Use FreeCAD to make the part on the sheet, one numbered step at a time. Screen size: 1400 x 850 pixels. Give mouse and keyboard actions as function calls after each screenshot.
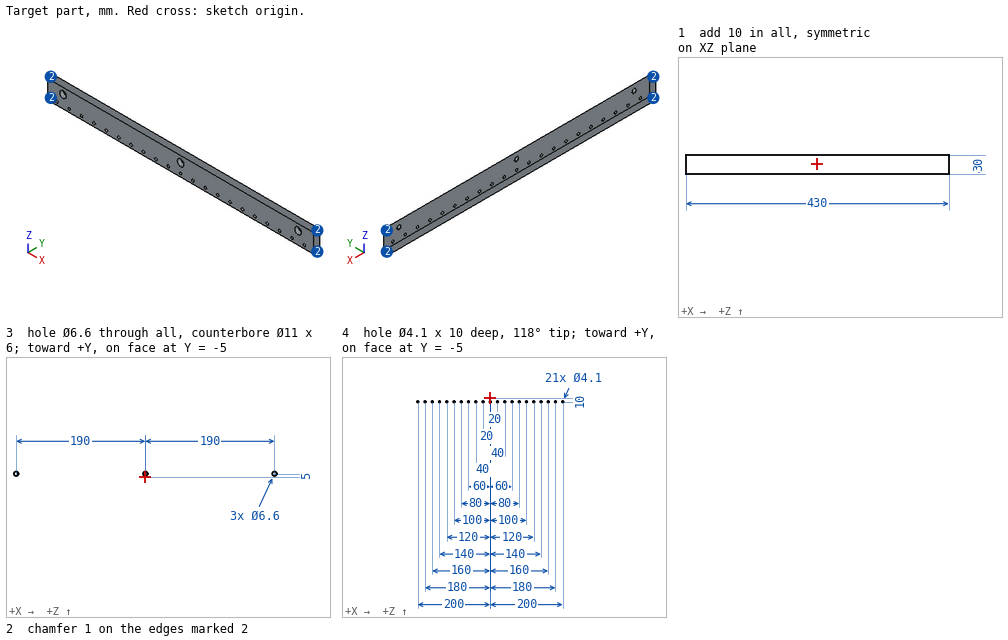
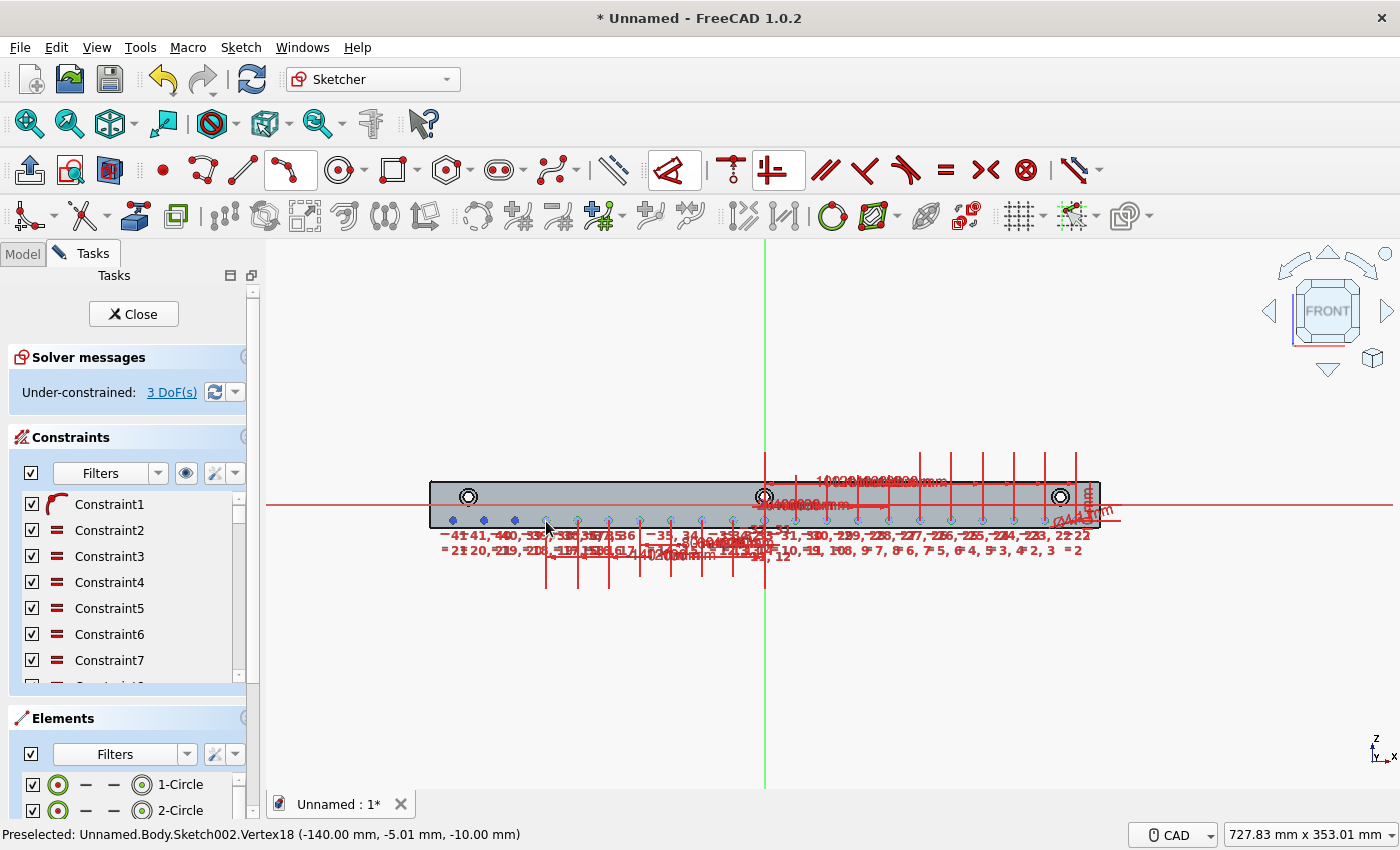
click(515, 521)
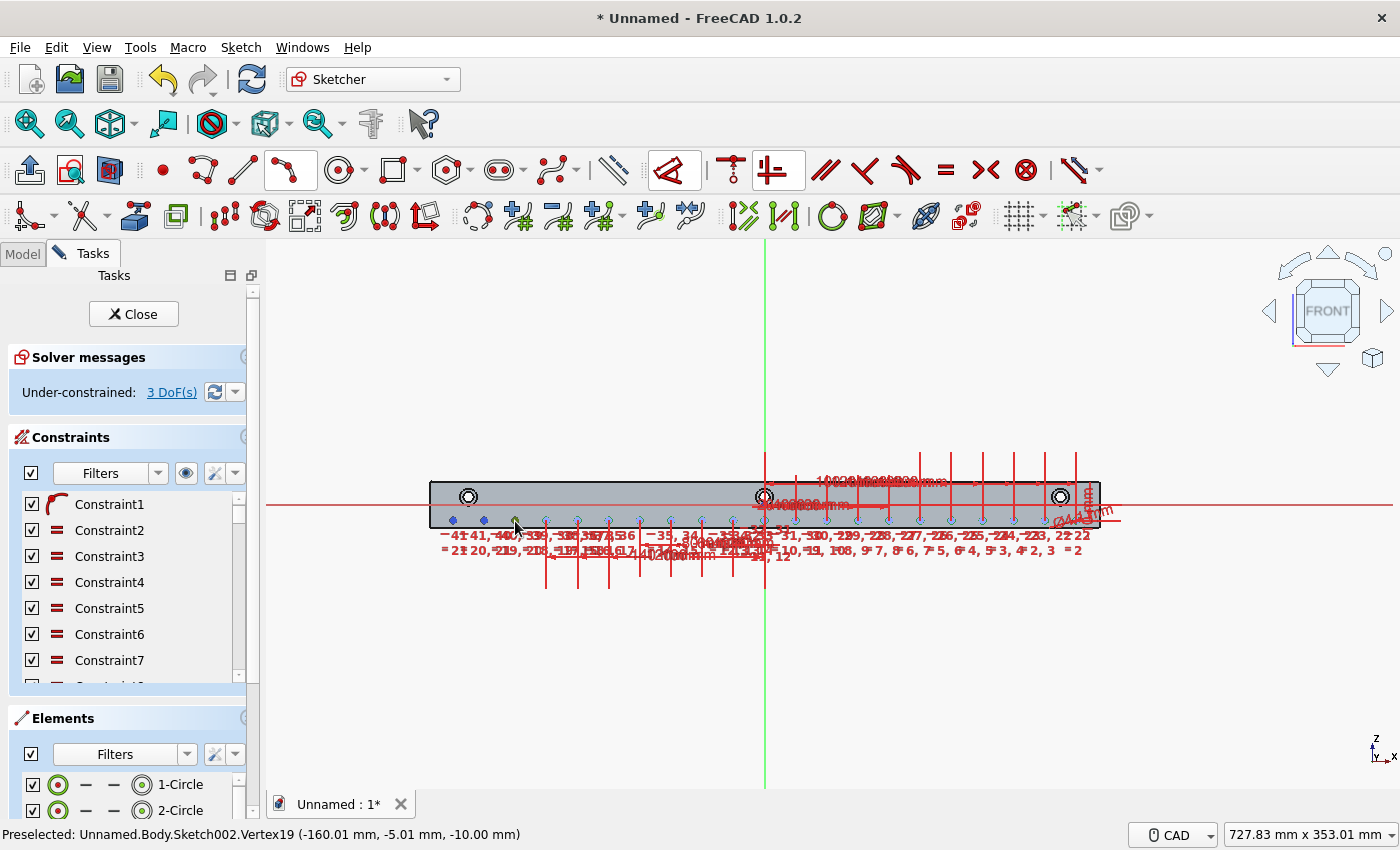
key(l)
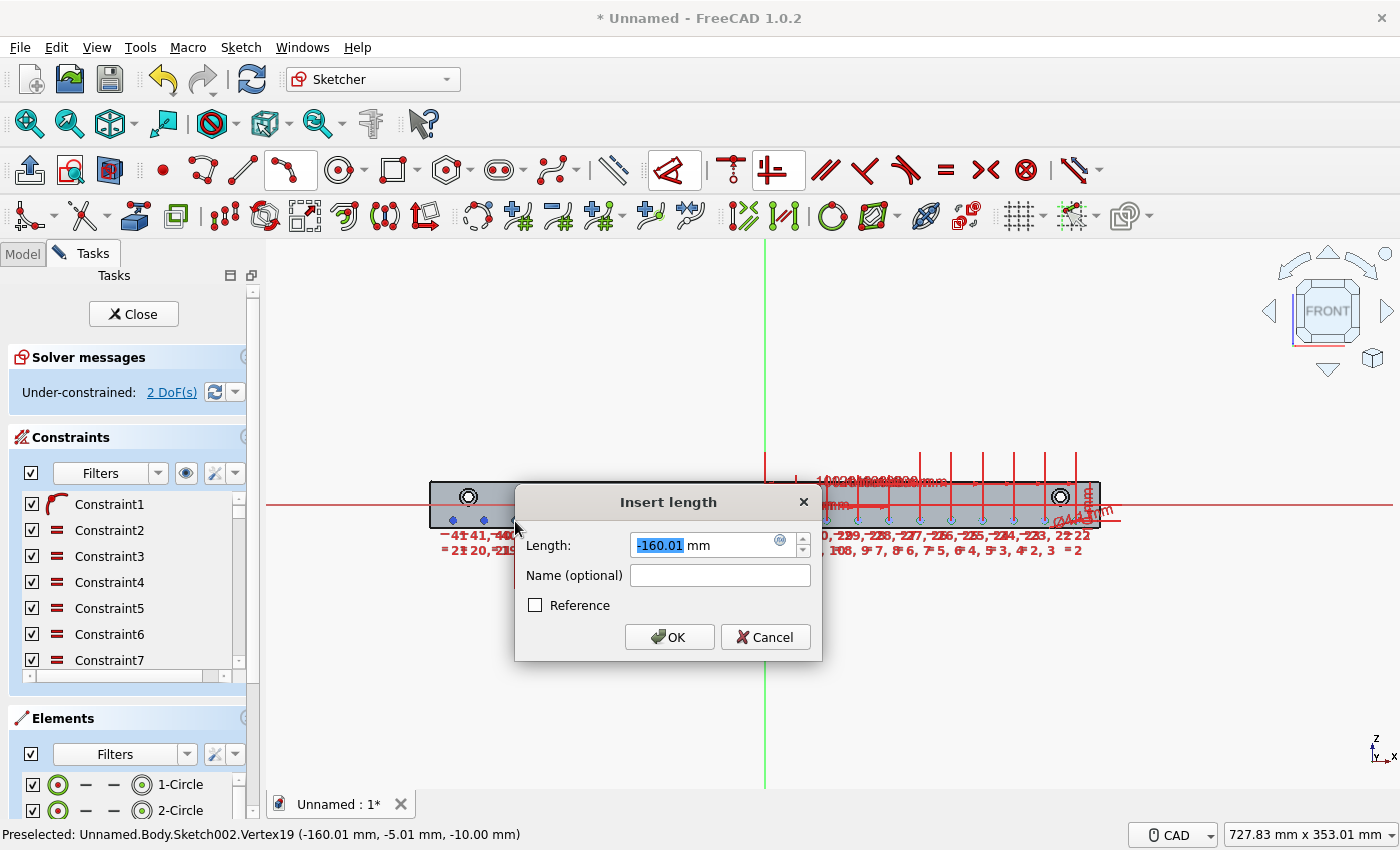
text(-160)
key(Return)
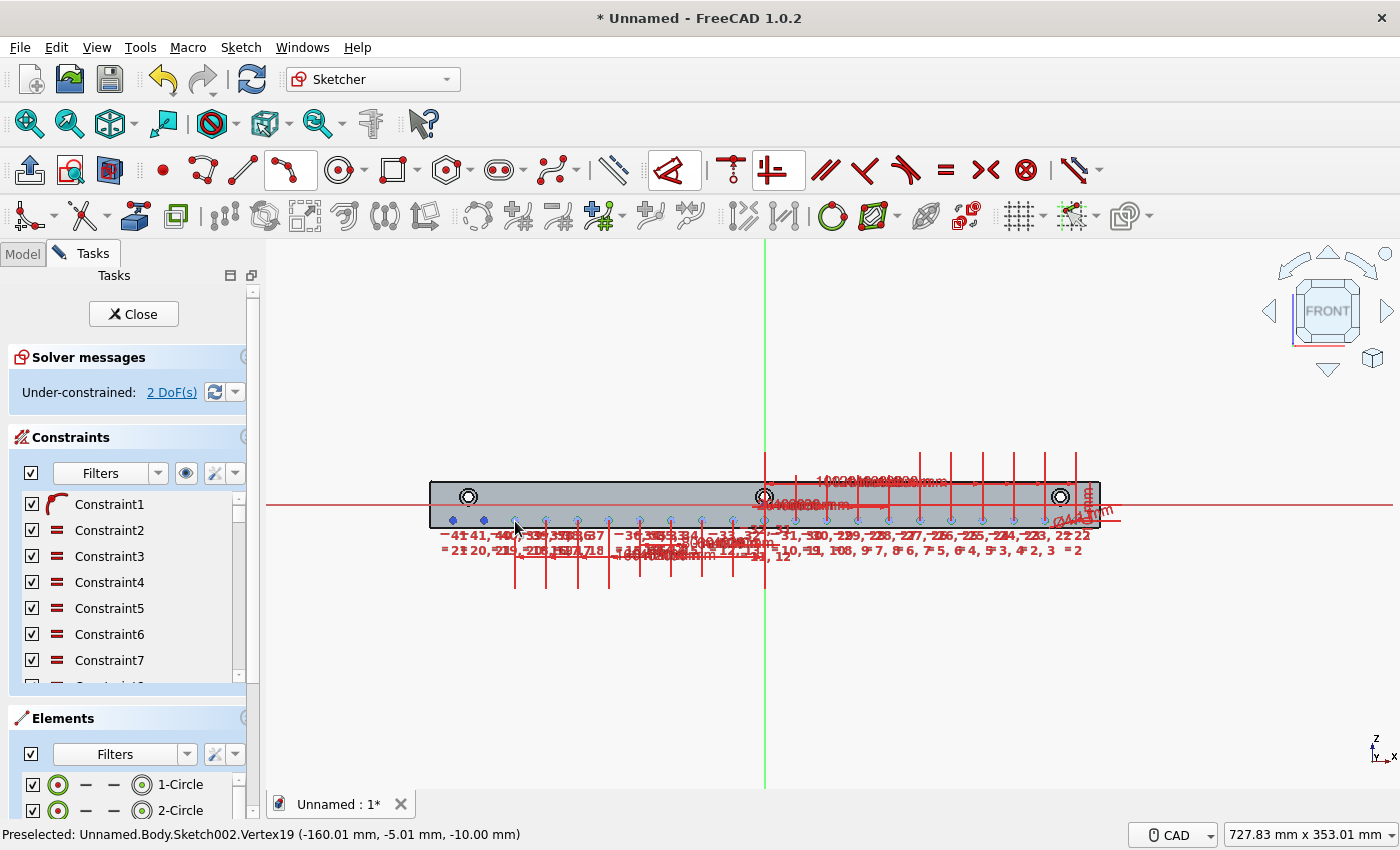
click(484, 521)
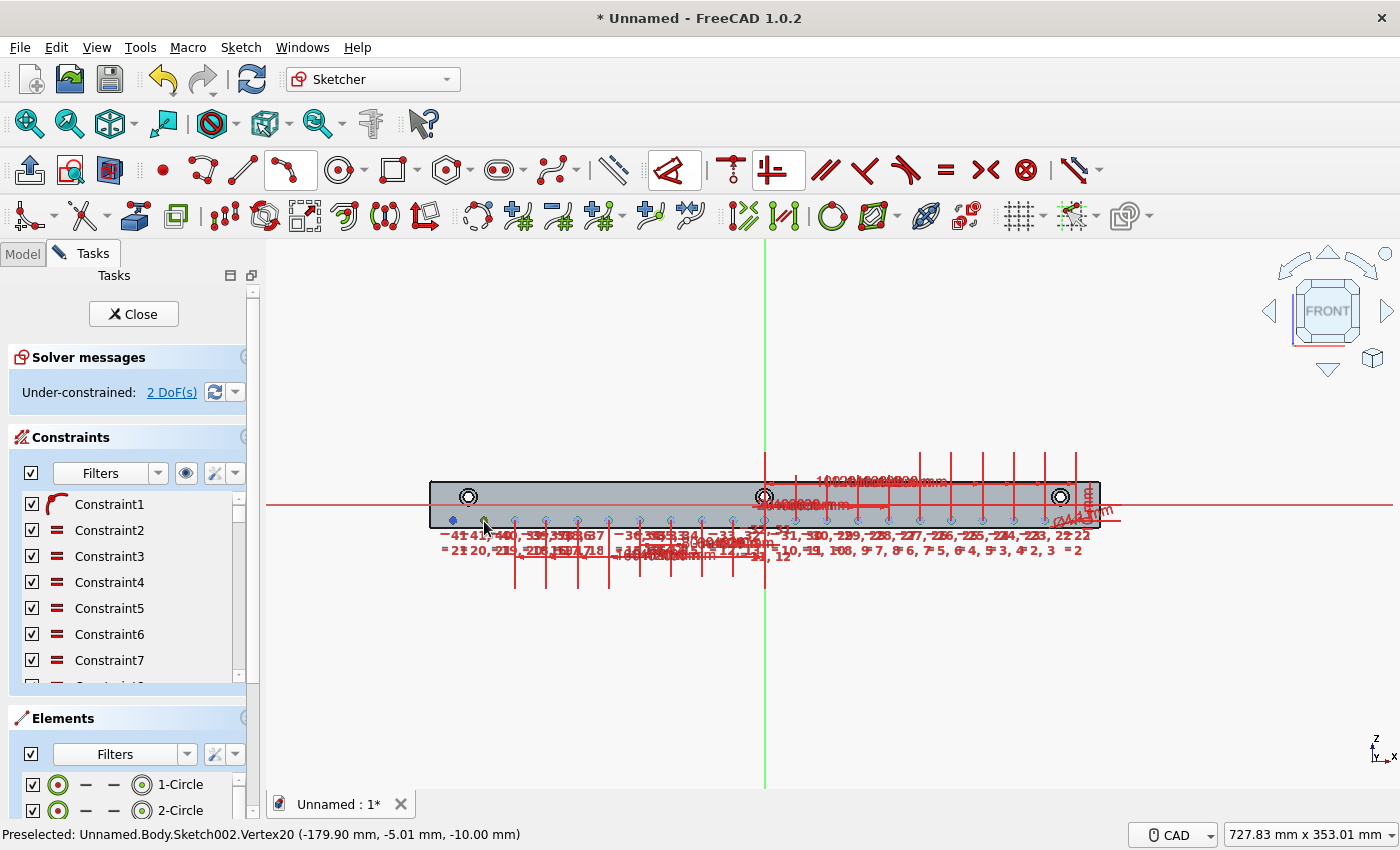
click(696, 170)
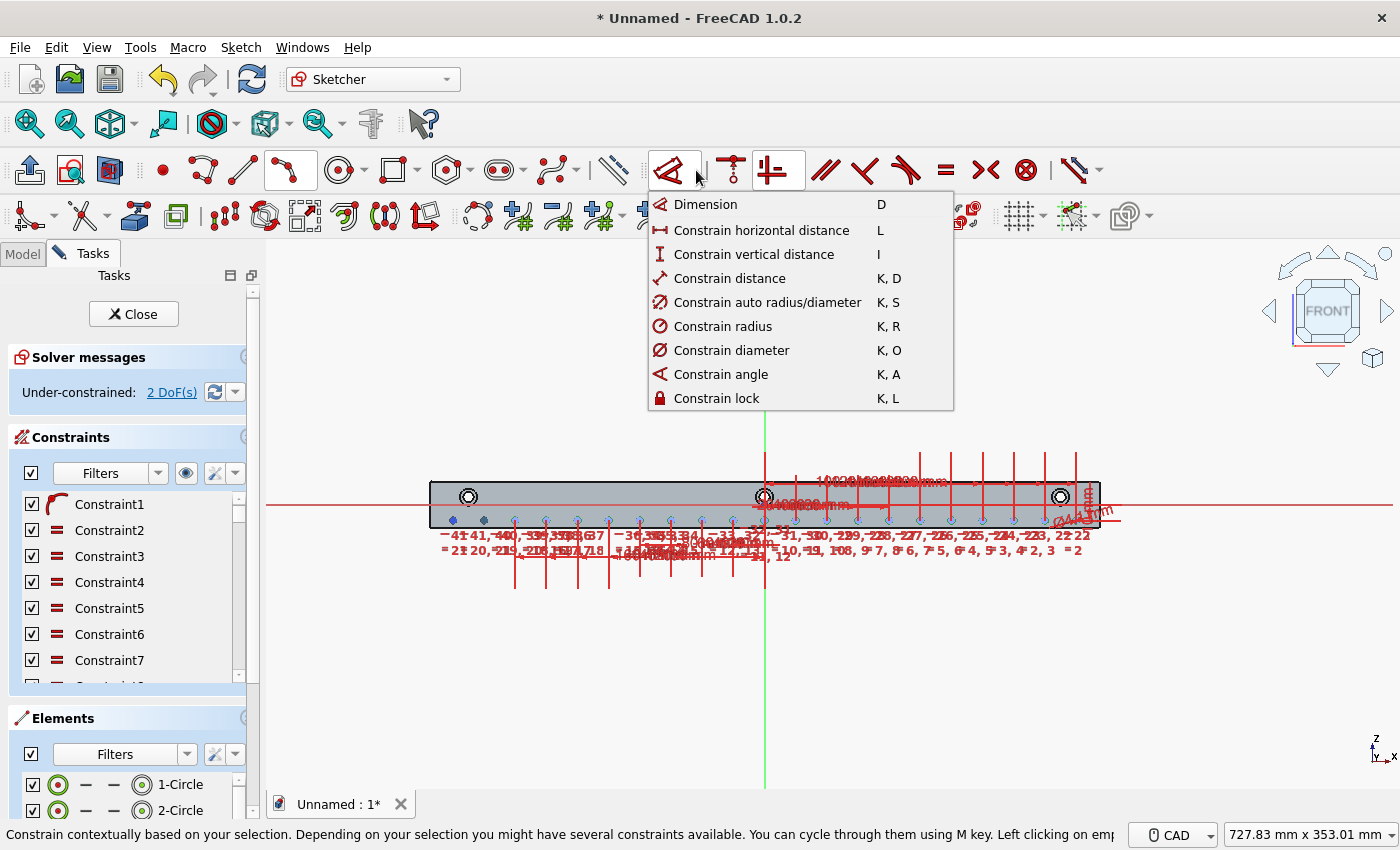
click(801, 230)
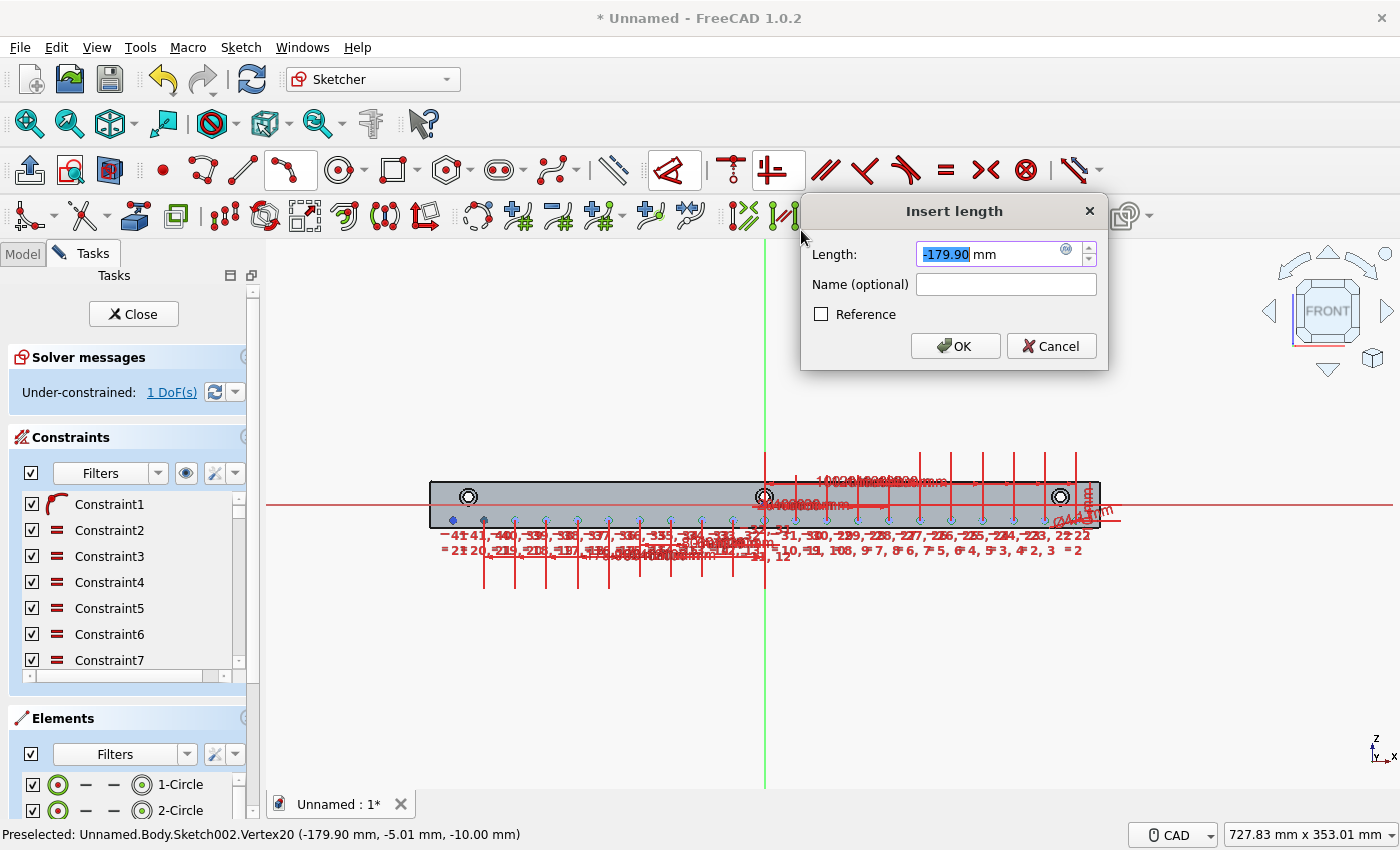
text(-180)
key(Return)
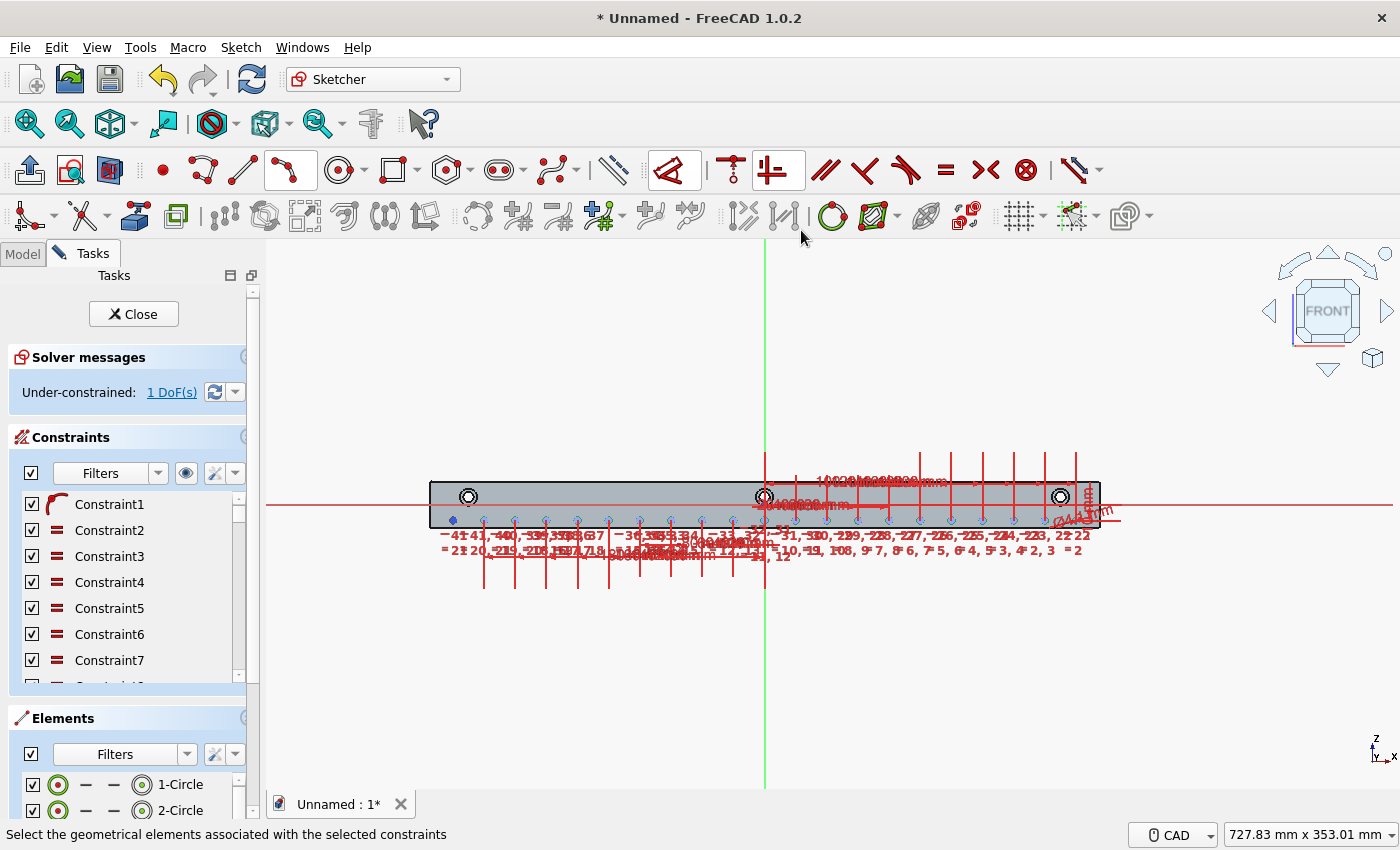
click(453, 521)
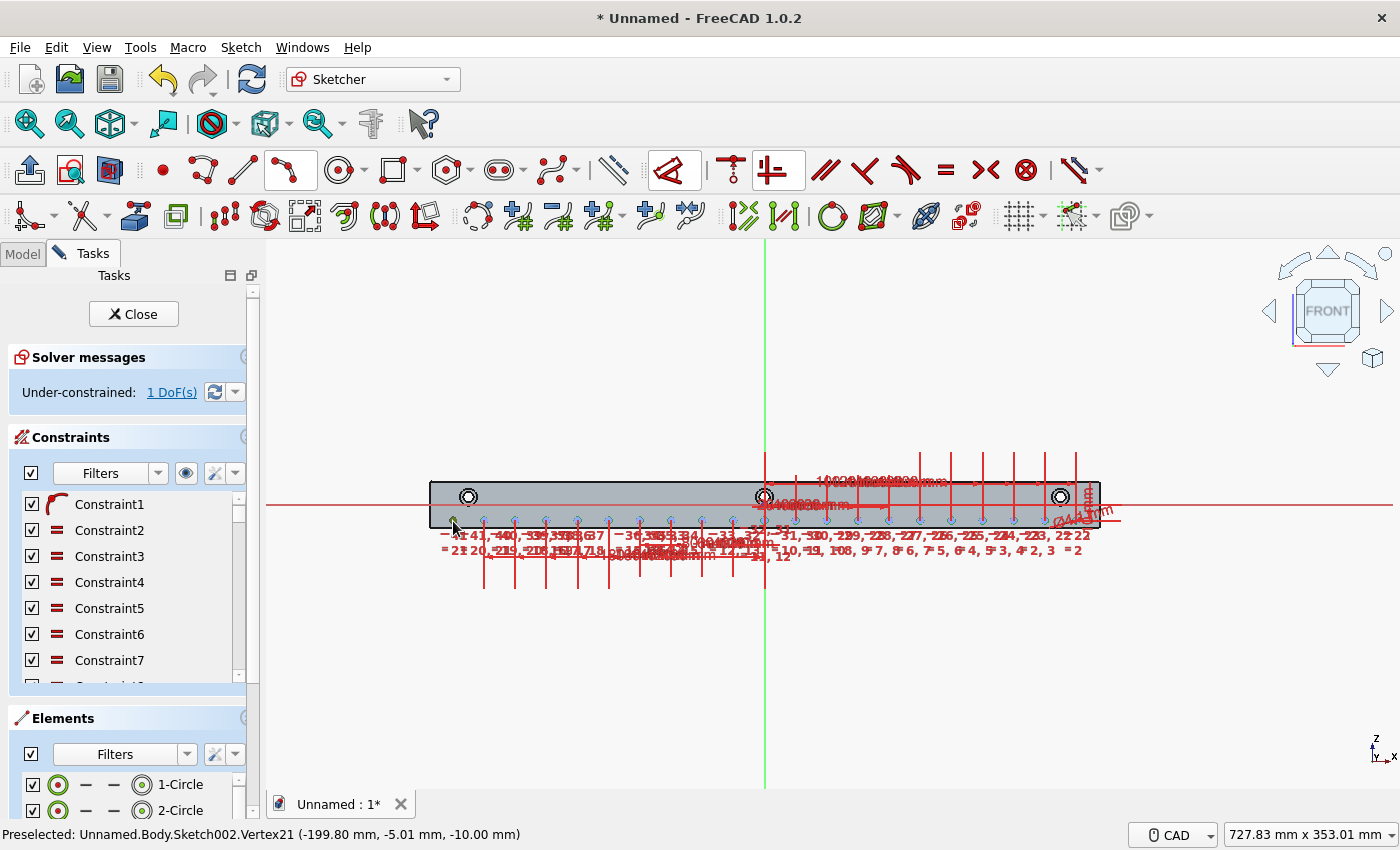
click(696, 170)